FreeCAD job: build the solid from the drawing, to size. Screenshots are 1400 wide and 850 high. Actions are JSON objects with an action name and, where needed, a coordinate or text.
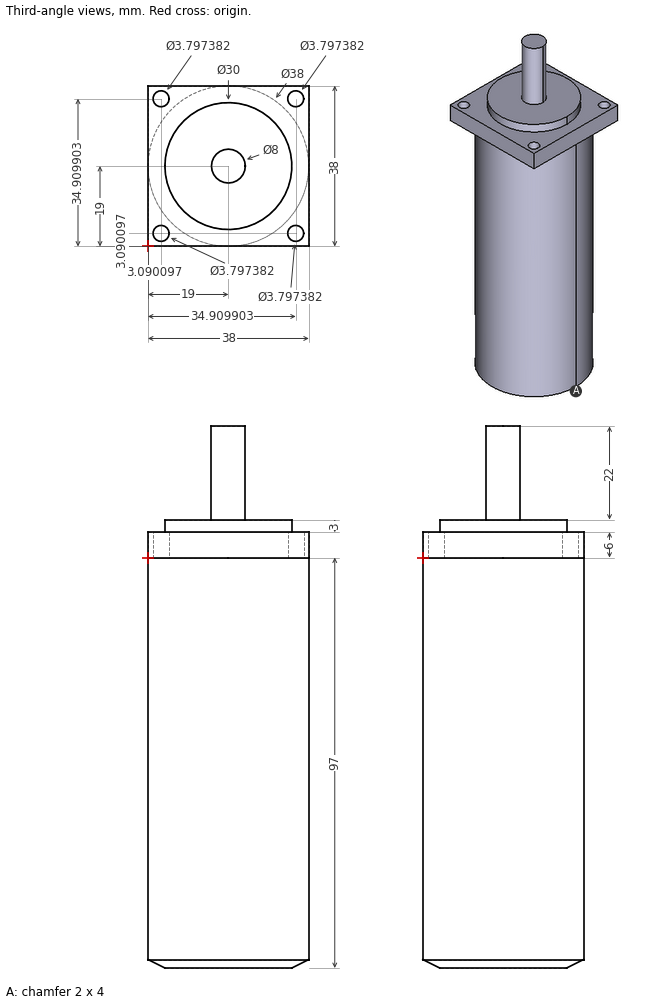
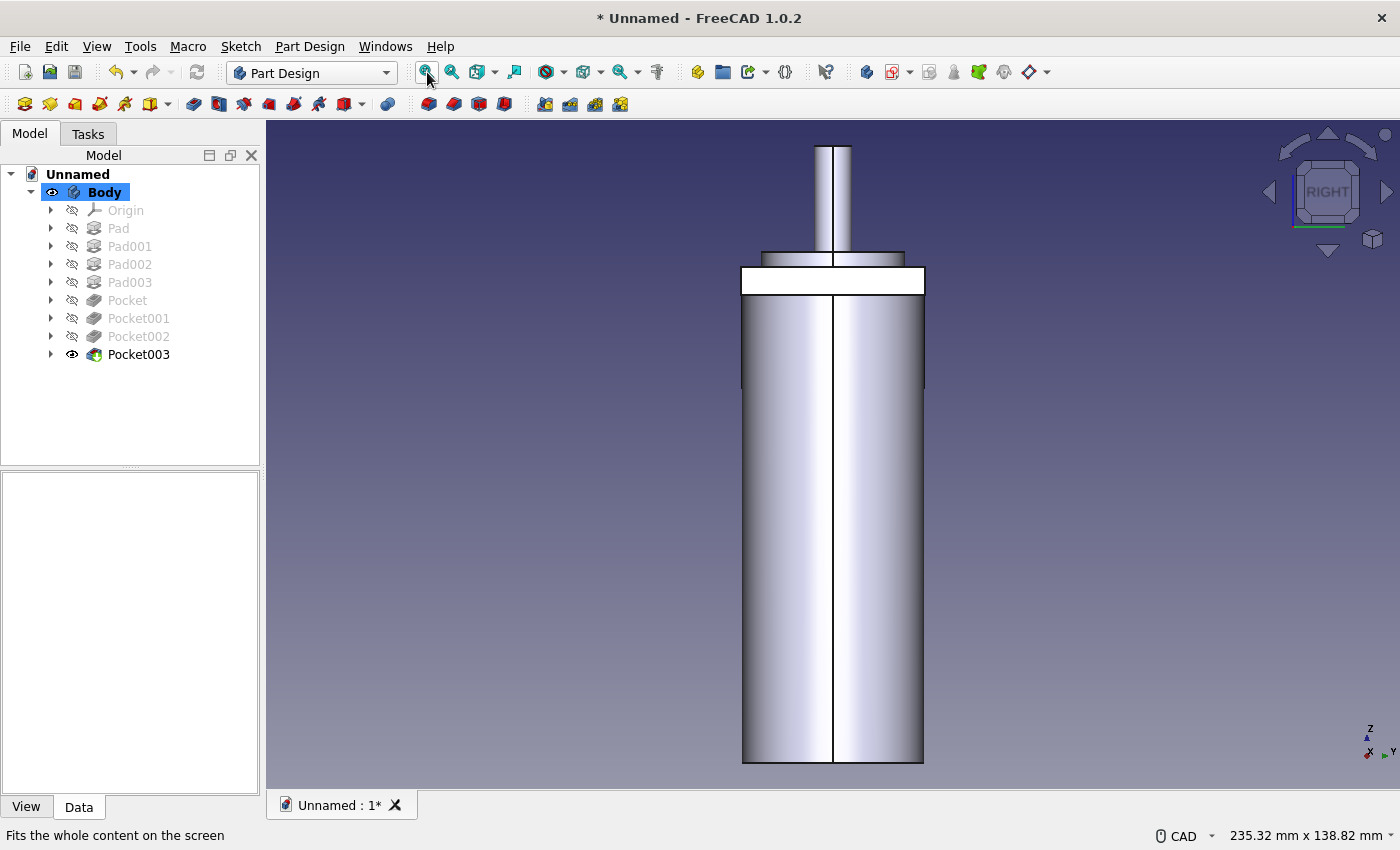
{"action": "key", "text": "5"}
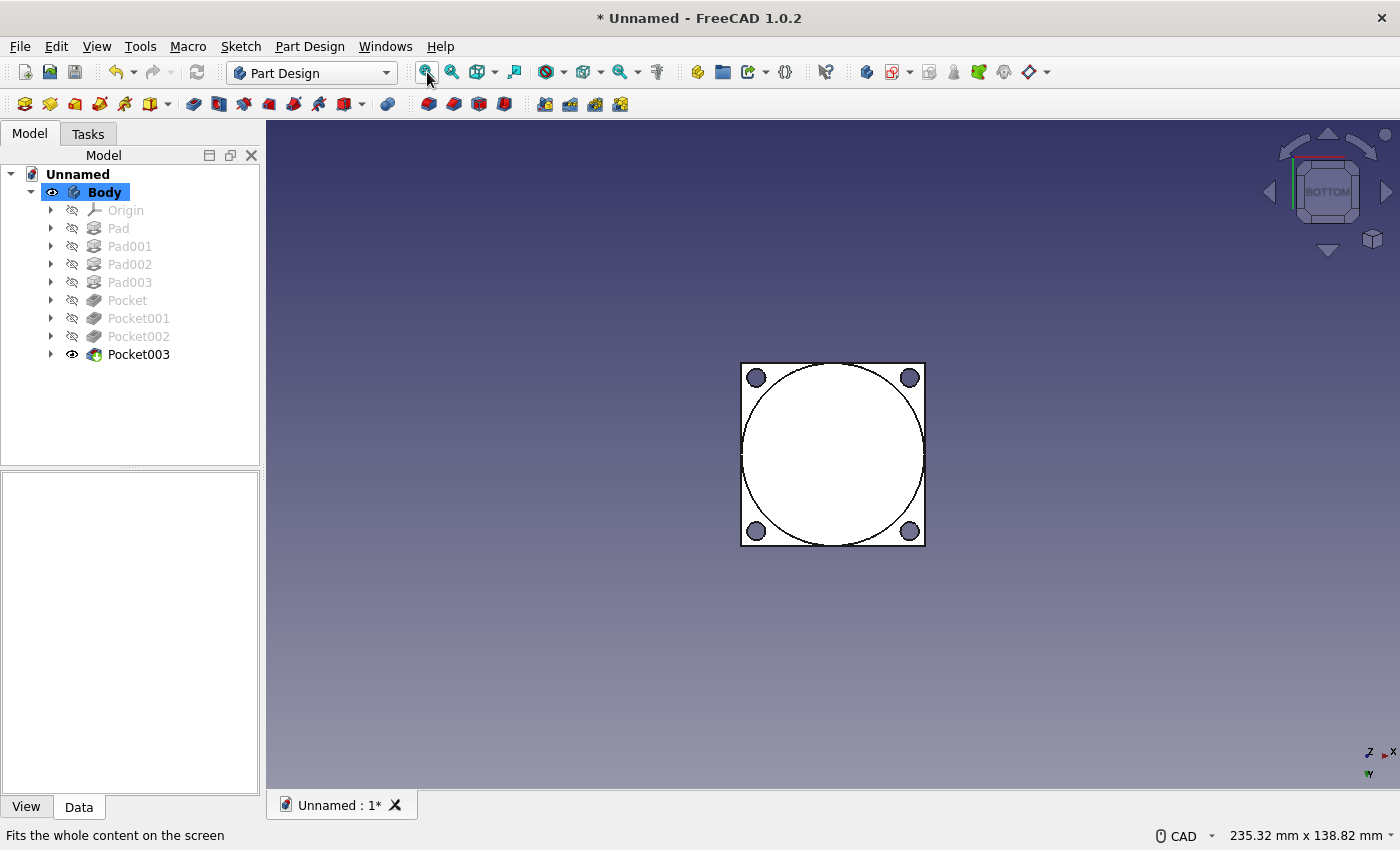
{"action": "left_click", "coordinate": [427, 72]}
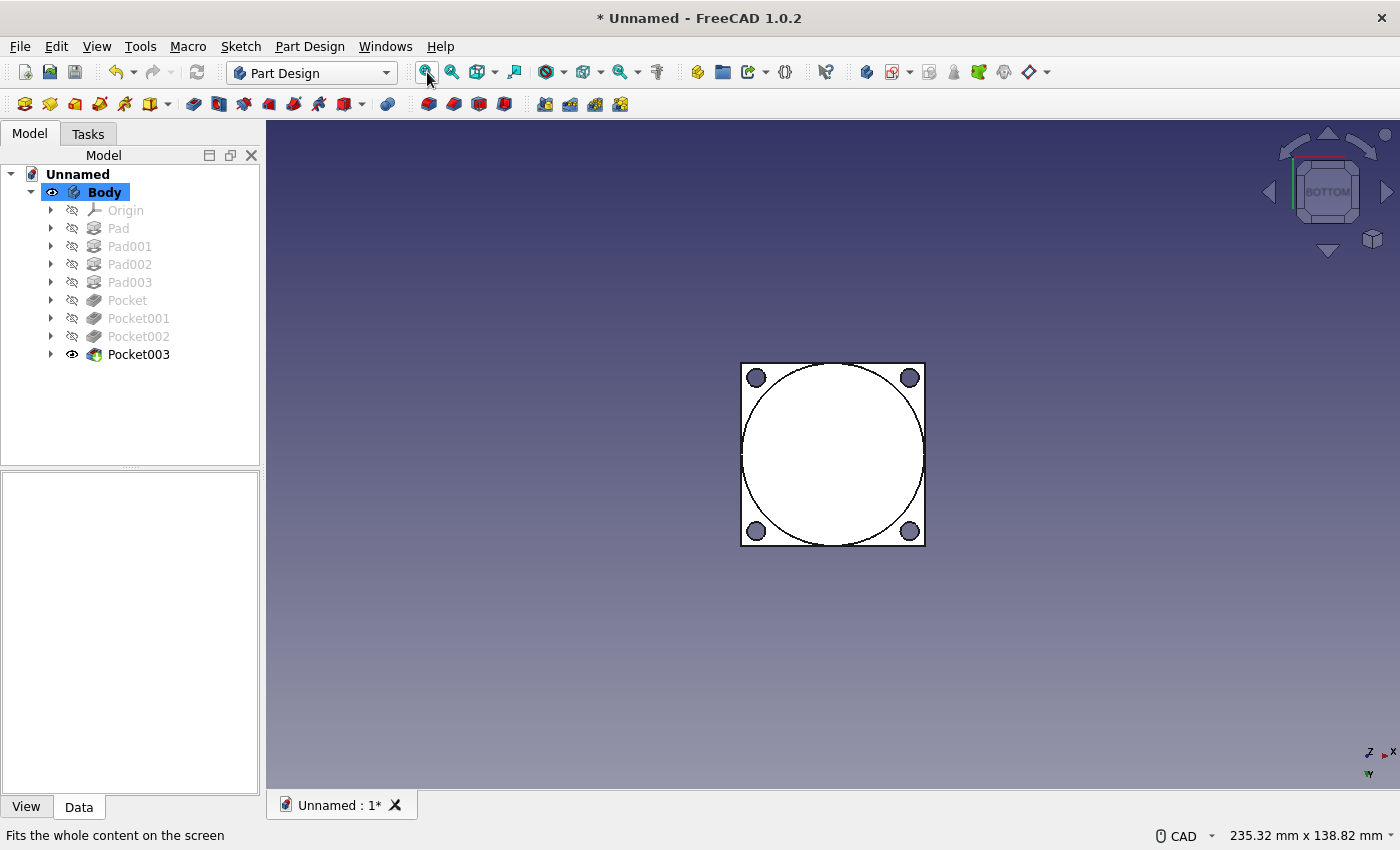
{"action": "left_click", "coordinate": [741, 453]}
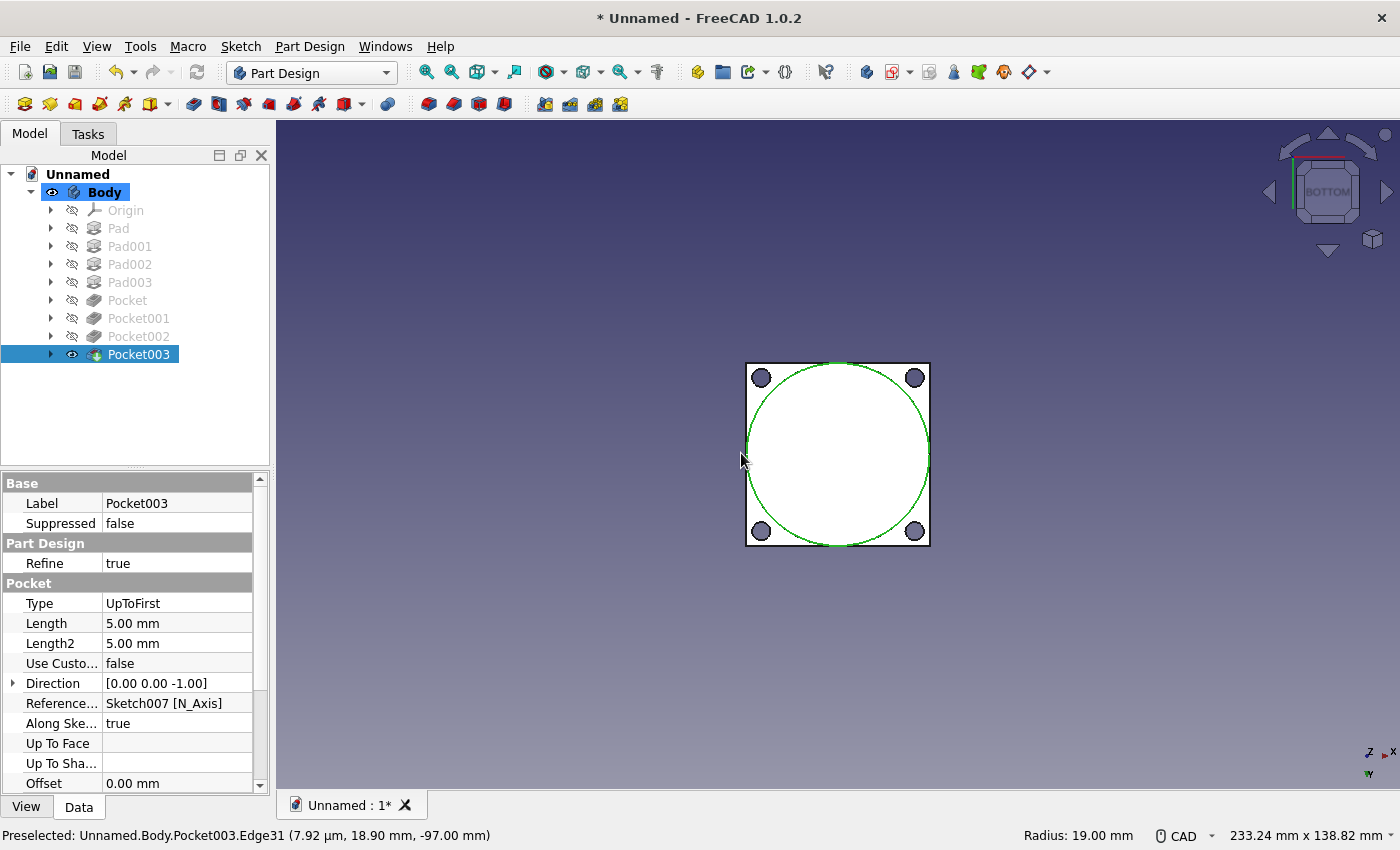
{"action": "left_click", "coordinate": [454, 104]}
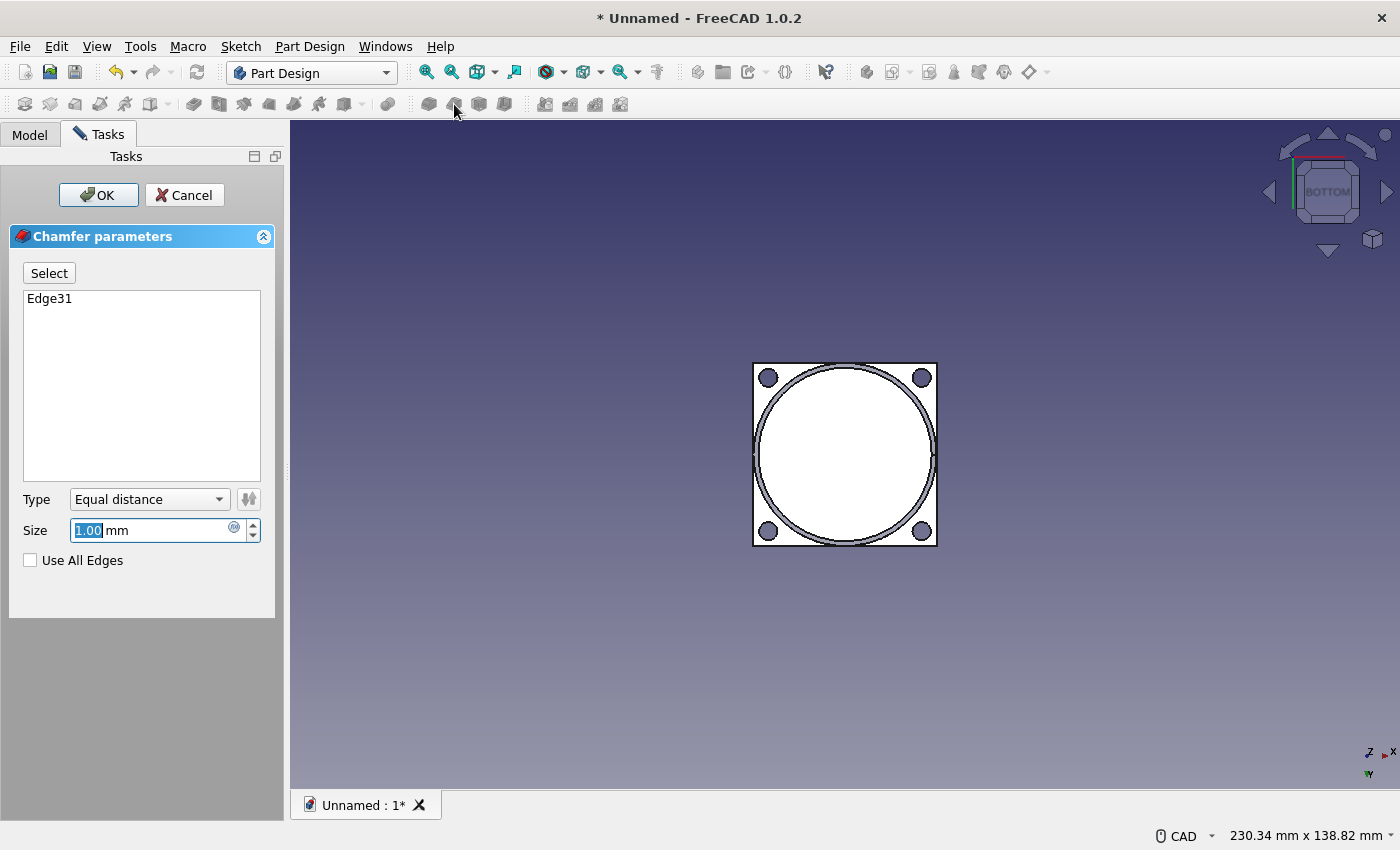
{"action": "type", "text": "2"}
{"action": "key", "text": "Tab"}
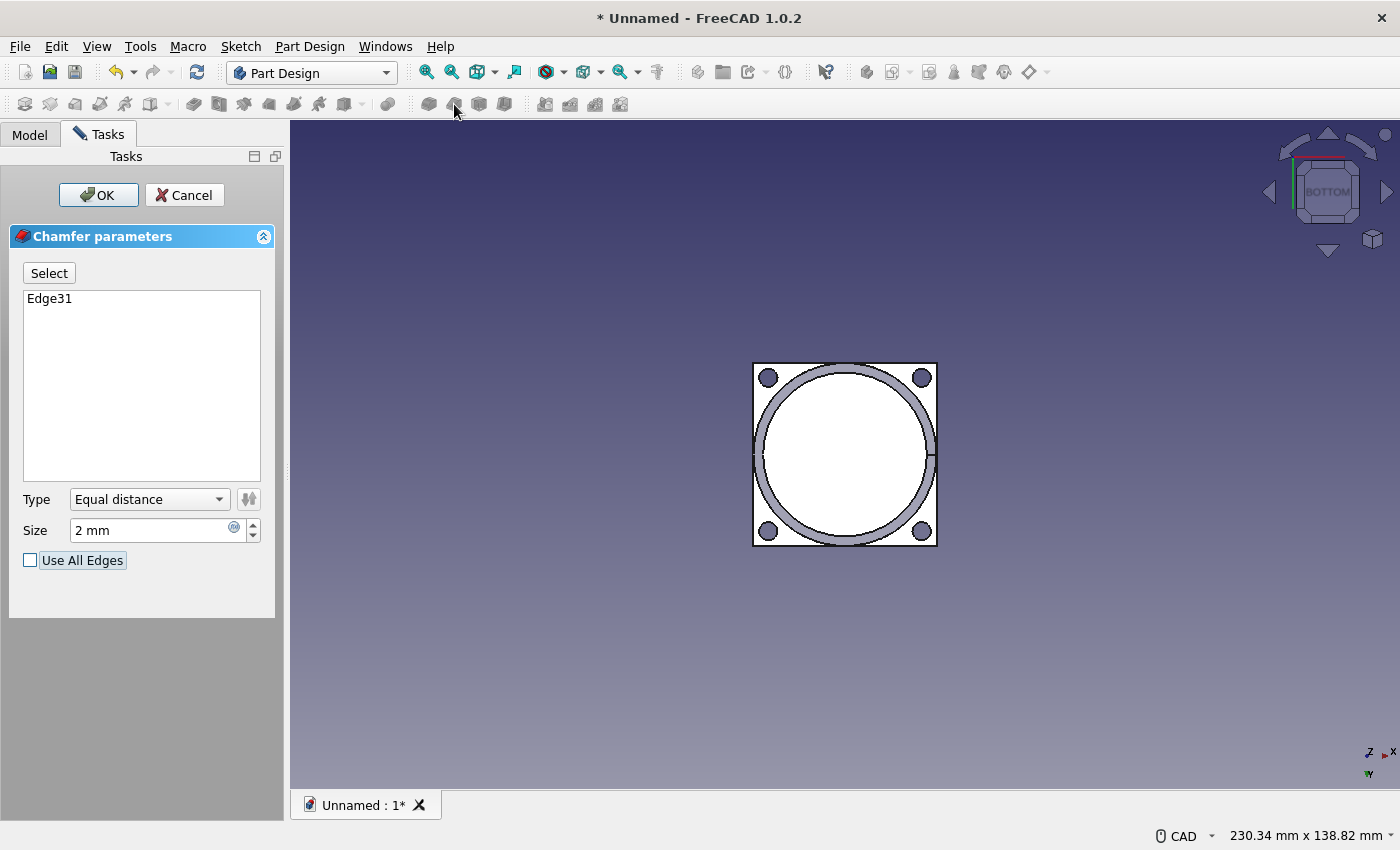
{"action": "left_click", "coordinate": [150, 500]}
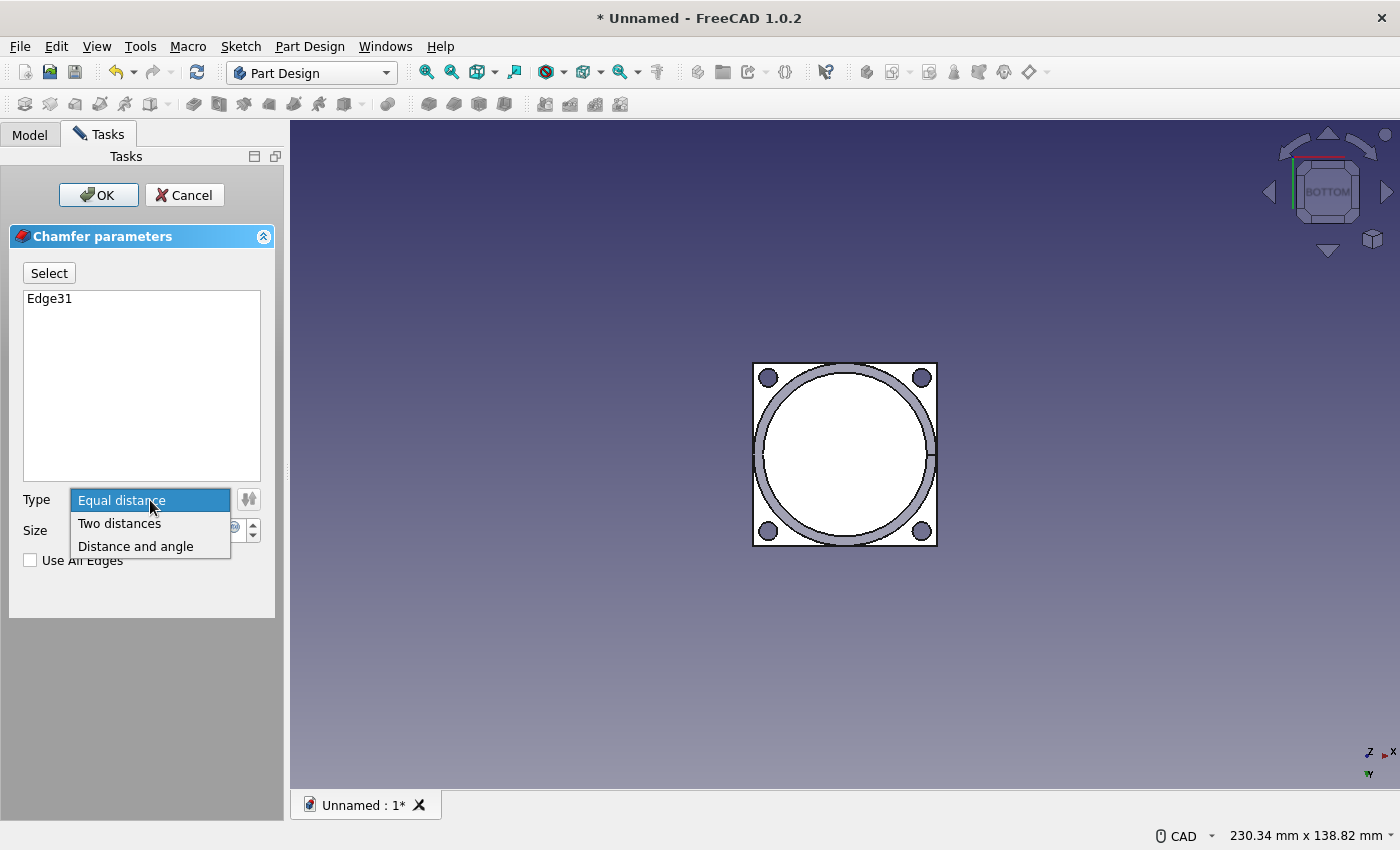
{"action": "left_click", "coordinate": [148, 524]}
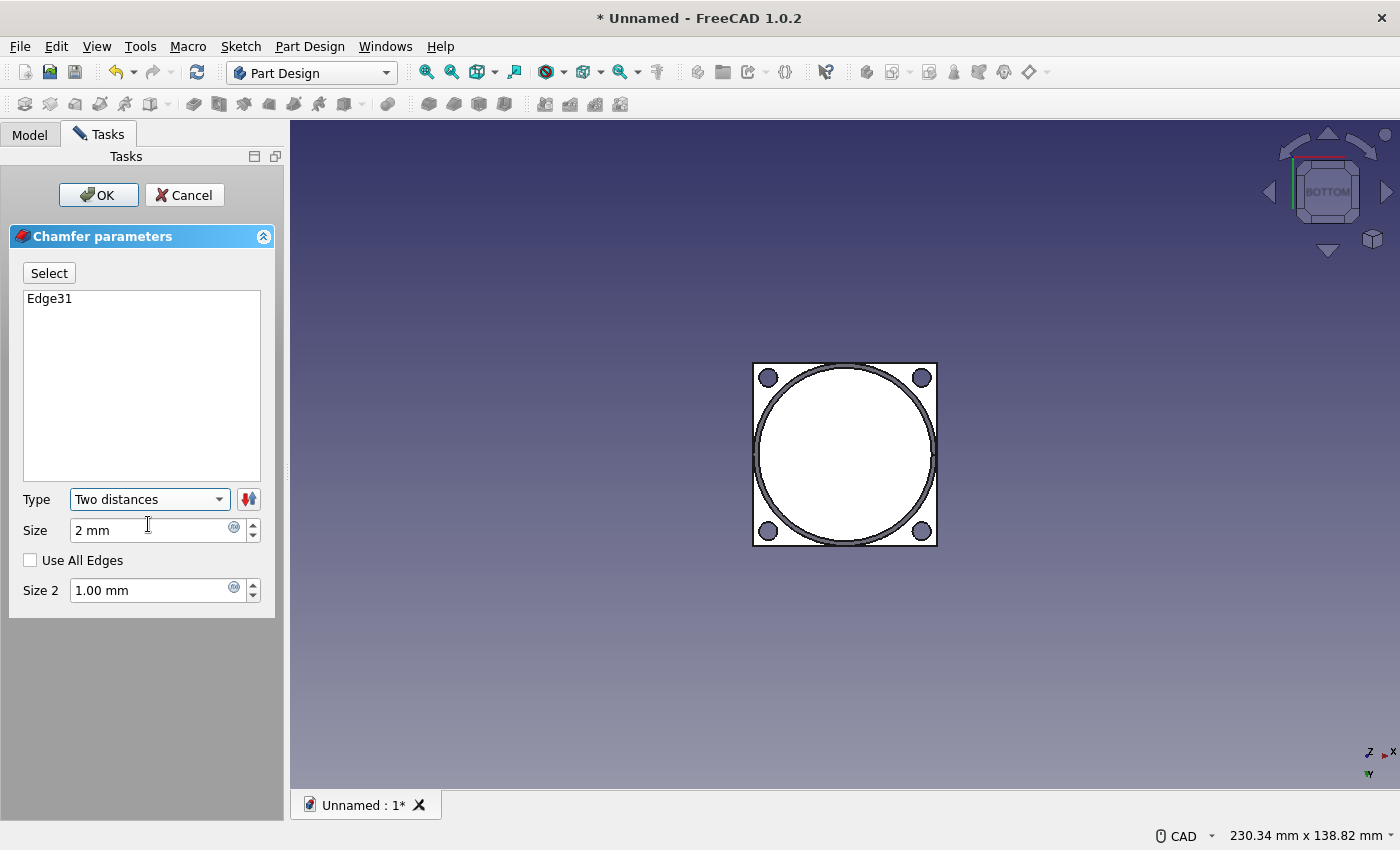
{"action": "triple_click", "coordinate": [158, 590]}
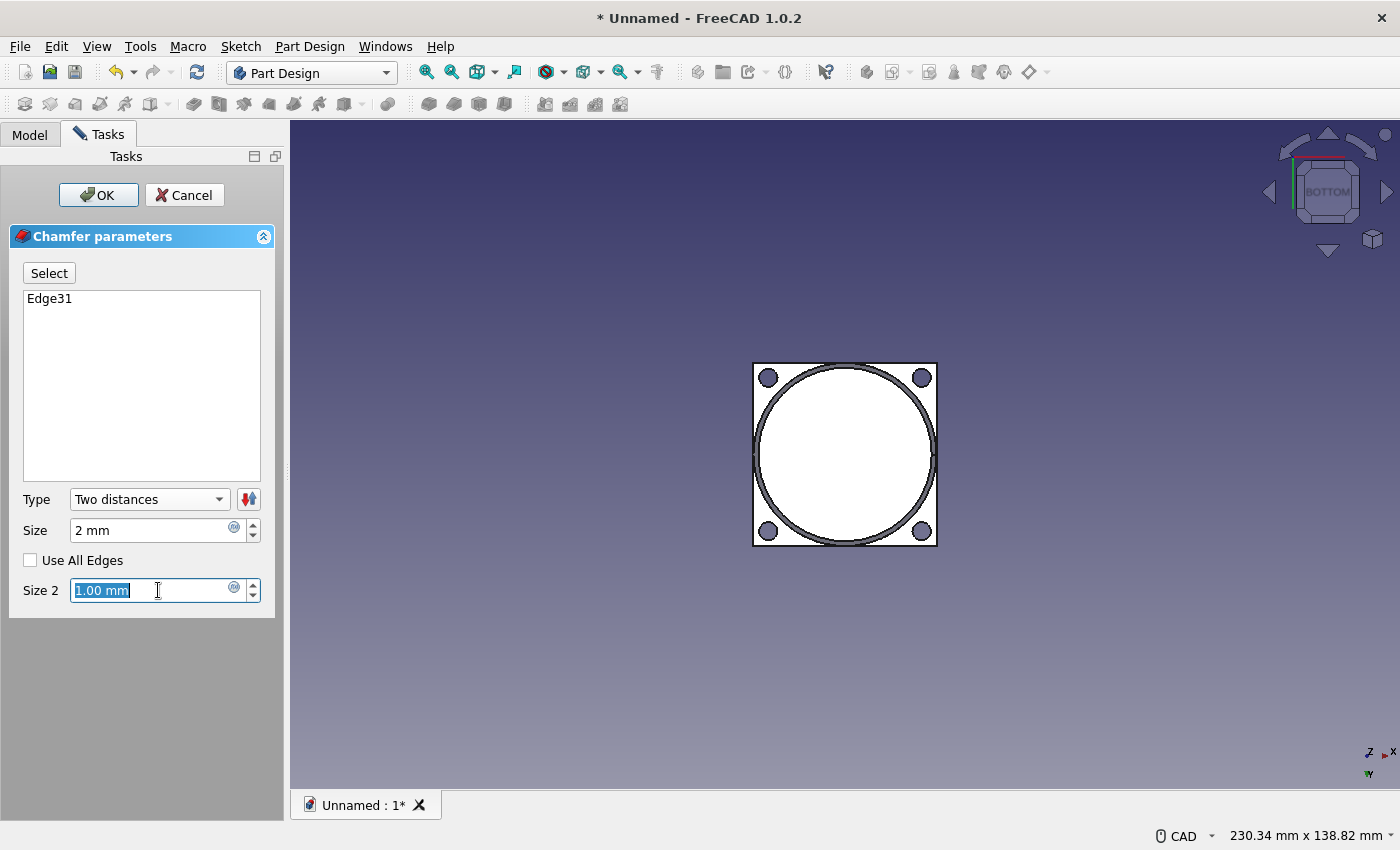
{"action": "type", "text": "4"}
{"action": "key", "text": "Tab"}